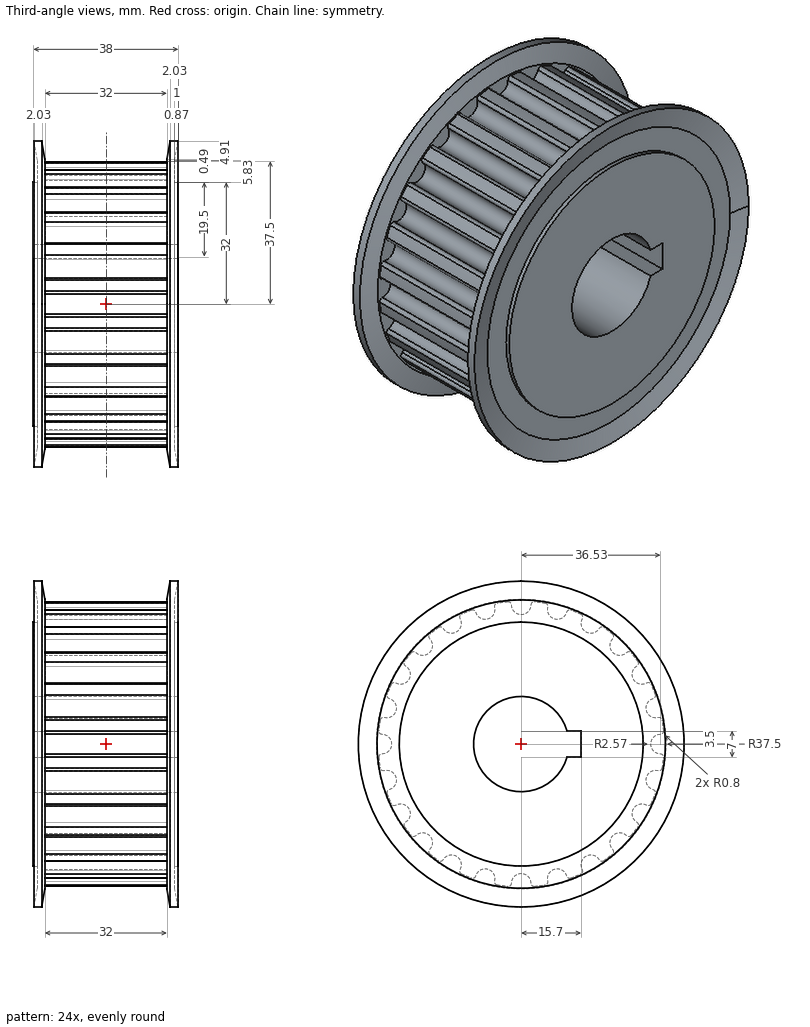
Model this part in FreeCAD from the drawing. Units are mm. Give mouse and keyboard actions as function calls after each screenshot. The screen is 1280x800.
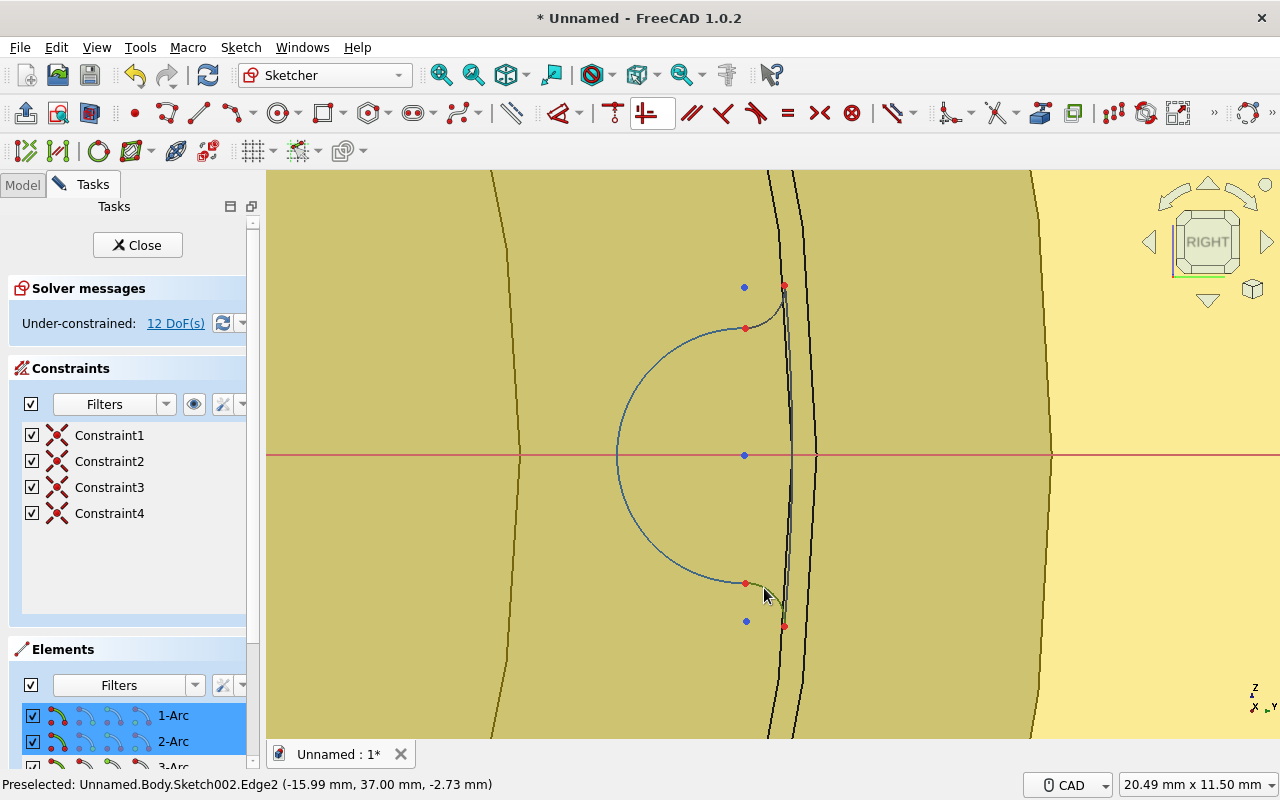
click(756, 114)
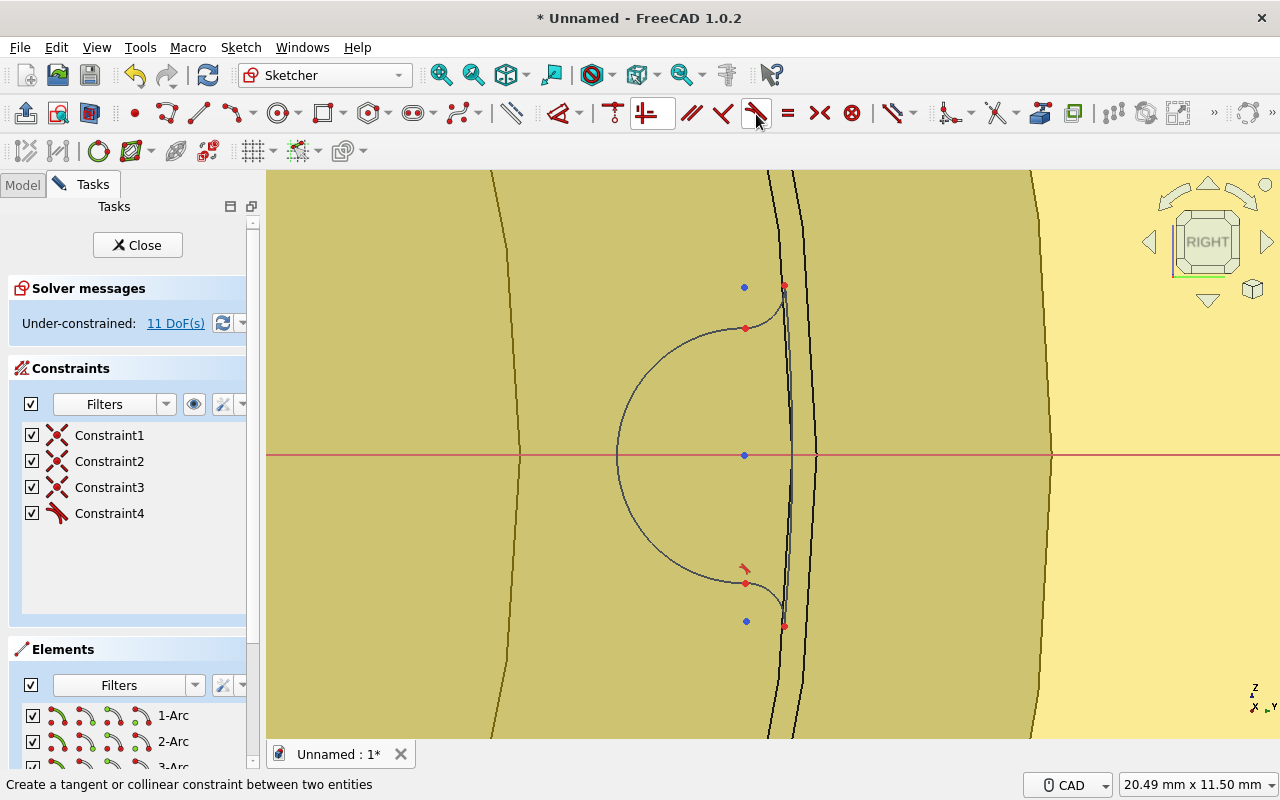
click(641, 381)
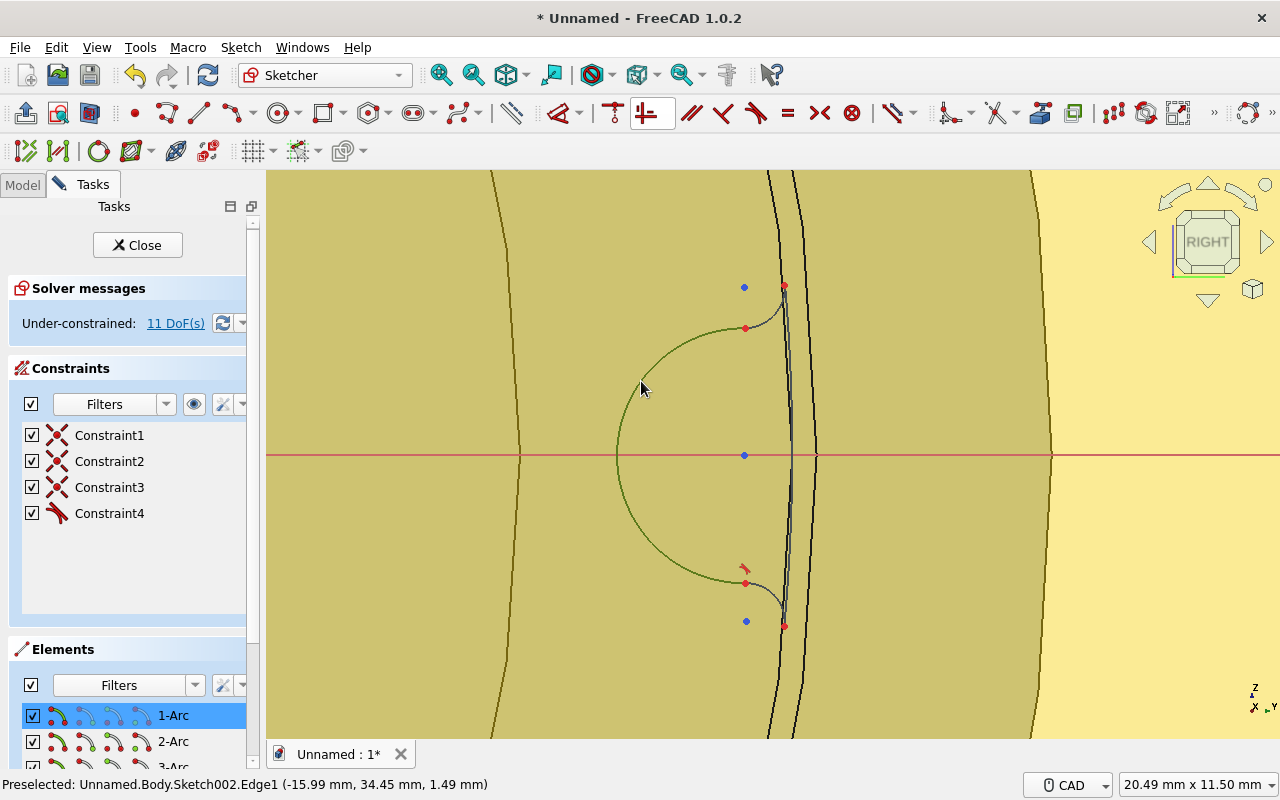
click(764, 323)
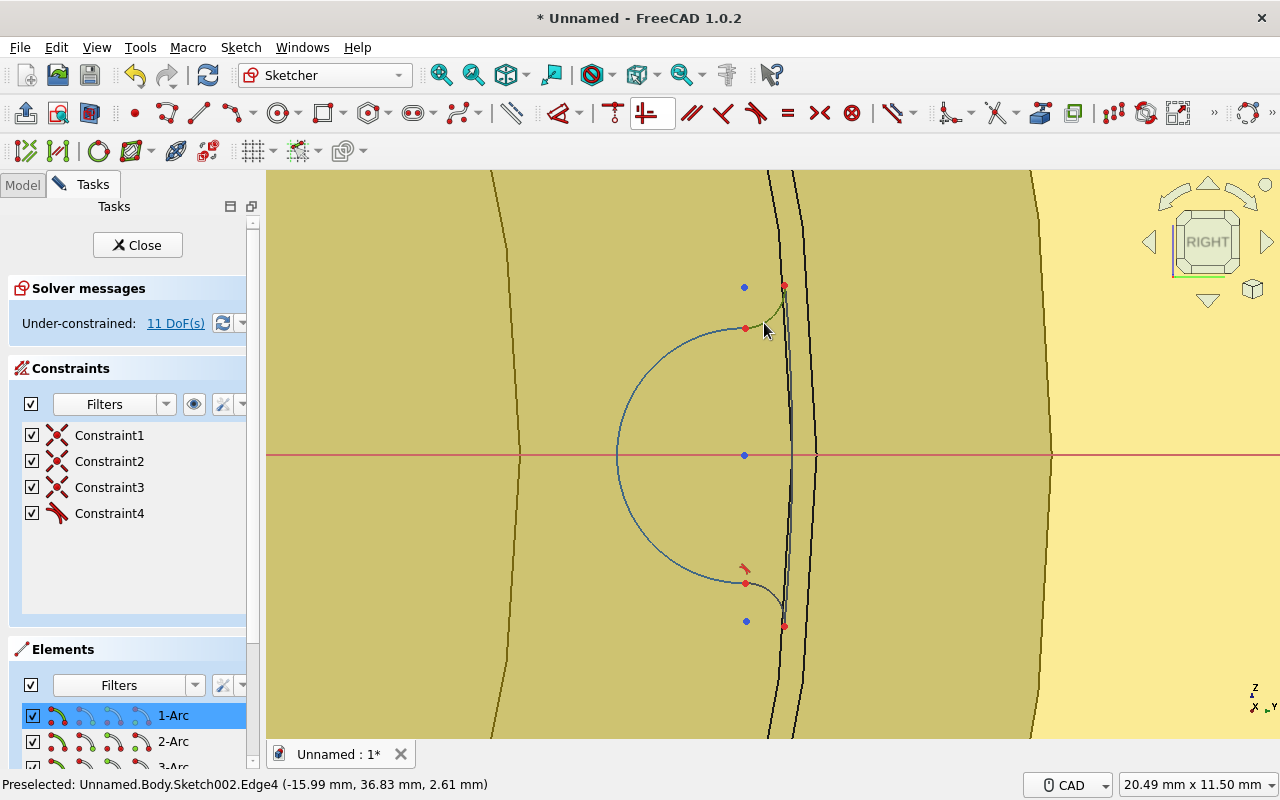
click(756, 114)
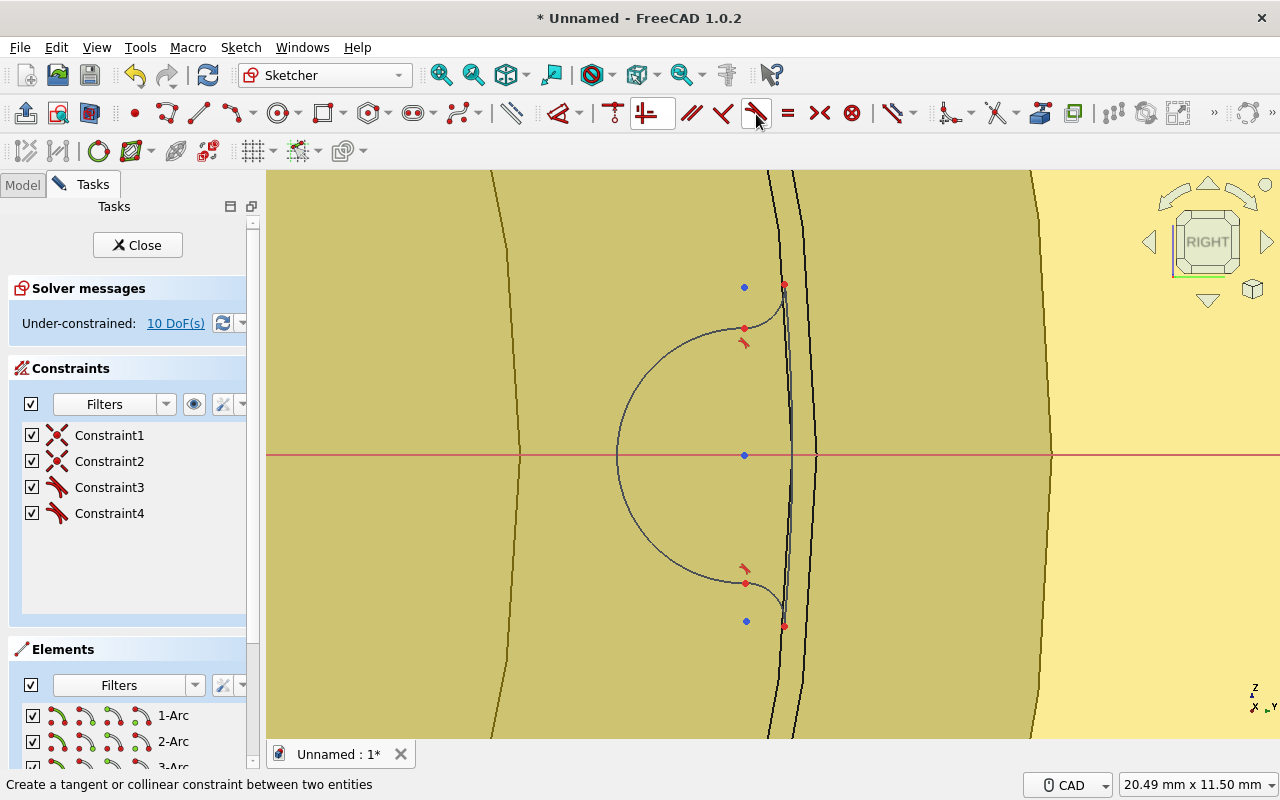
click(765, 588)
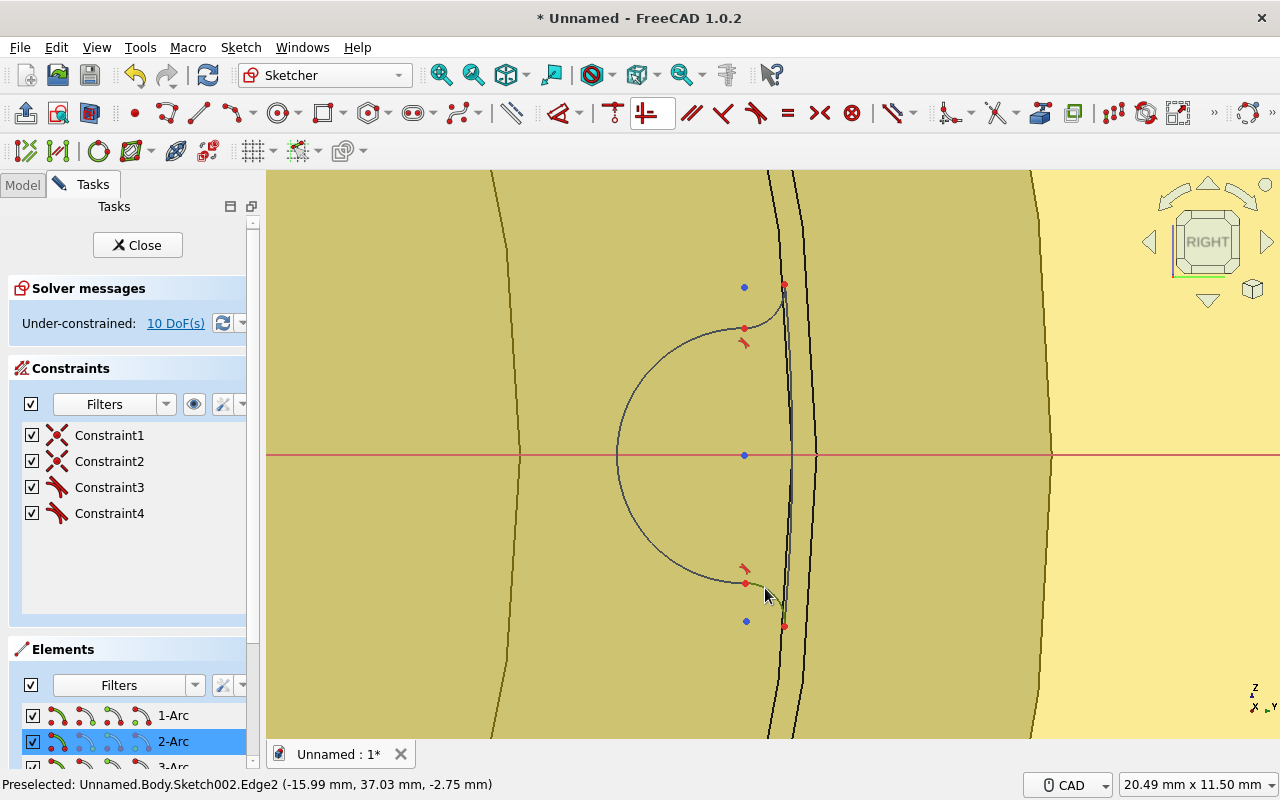
click(791, 524)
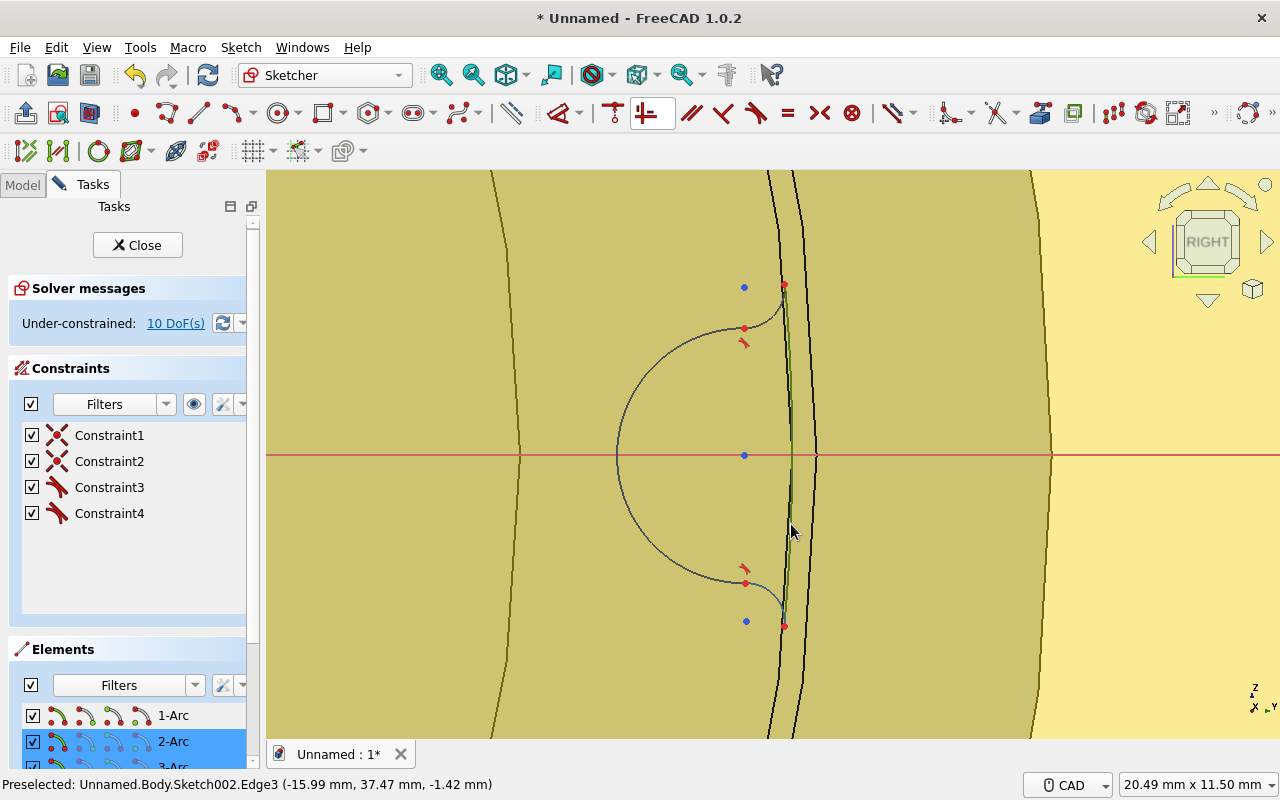
click(756, 114)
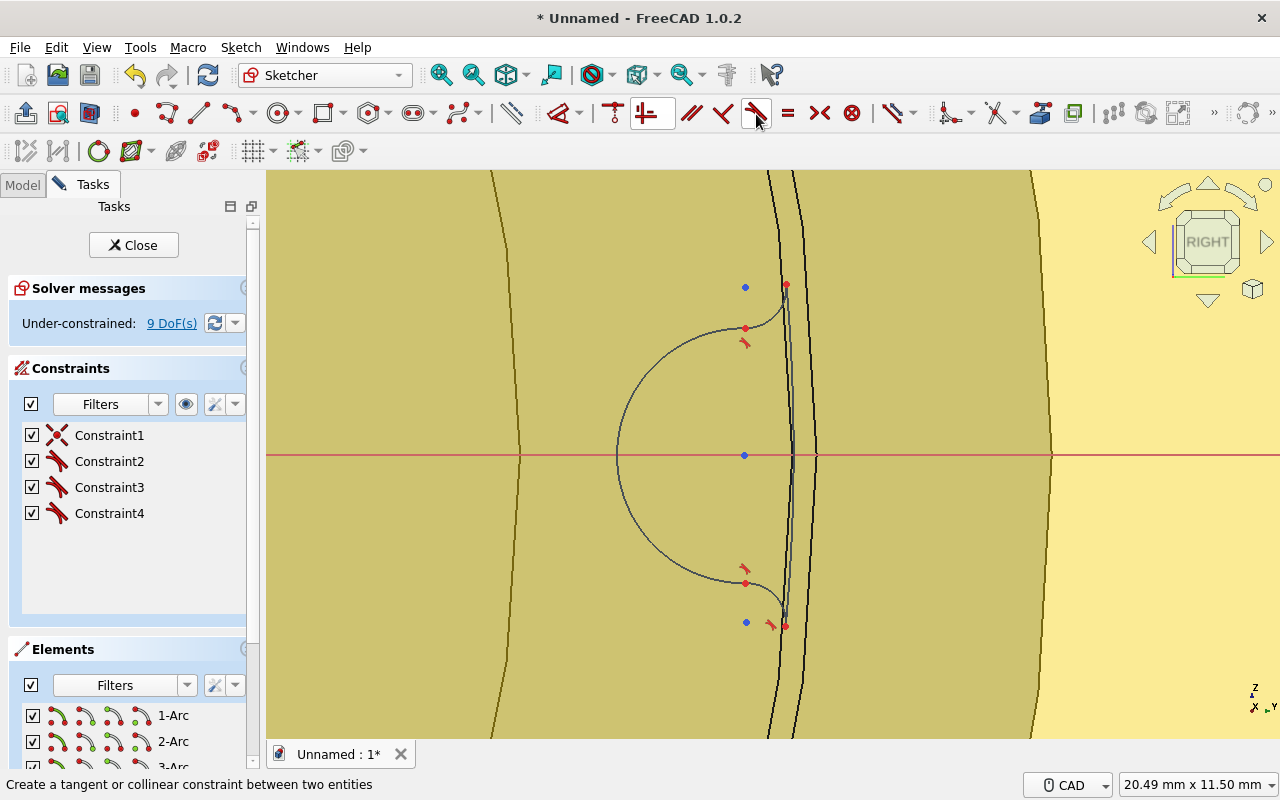
click(792, 524)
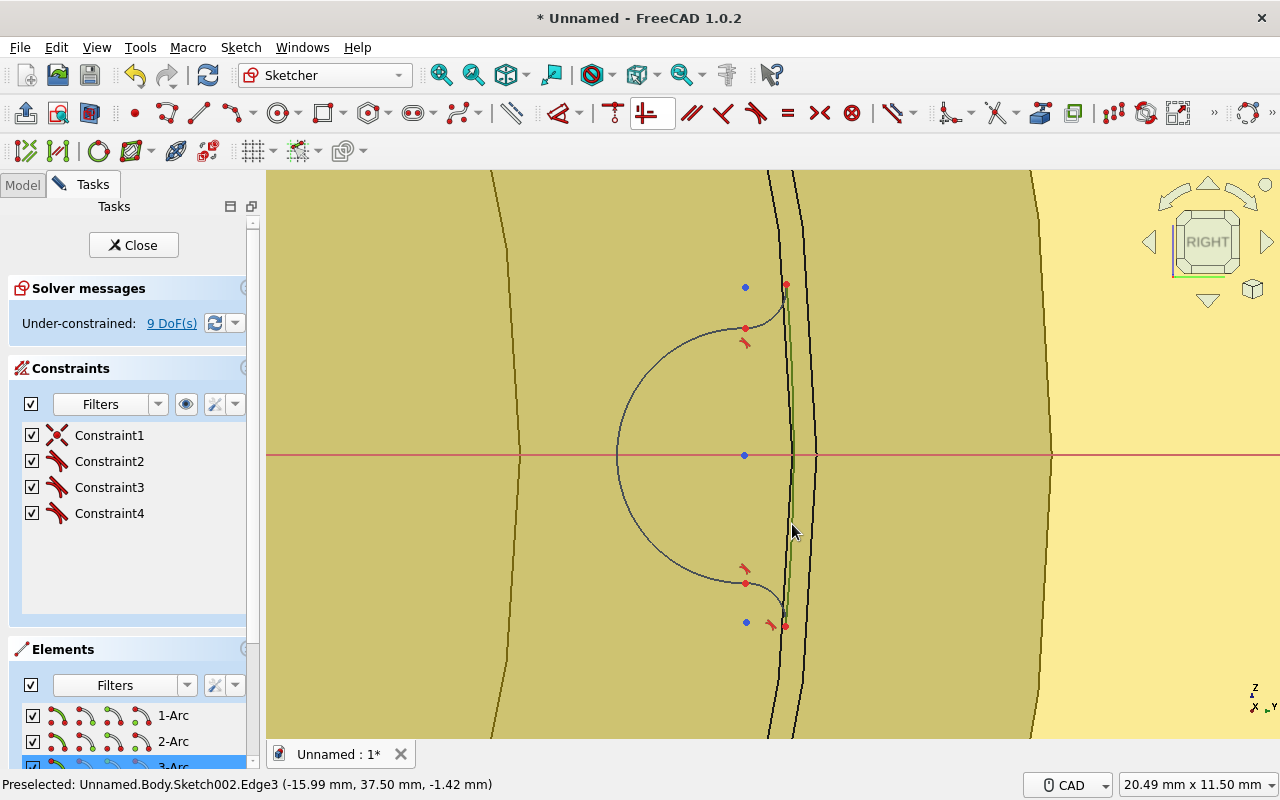
click(765, 324)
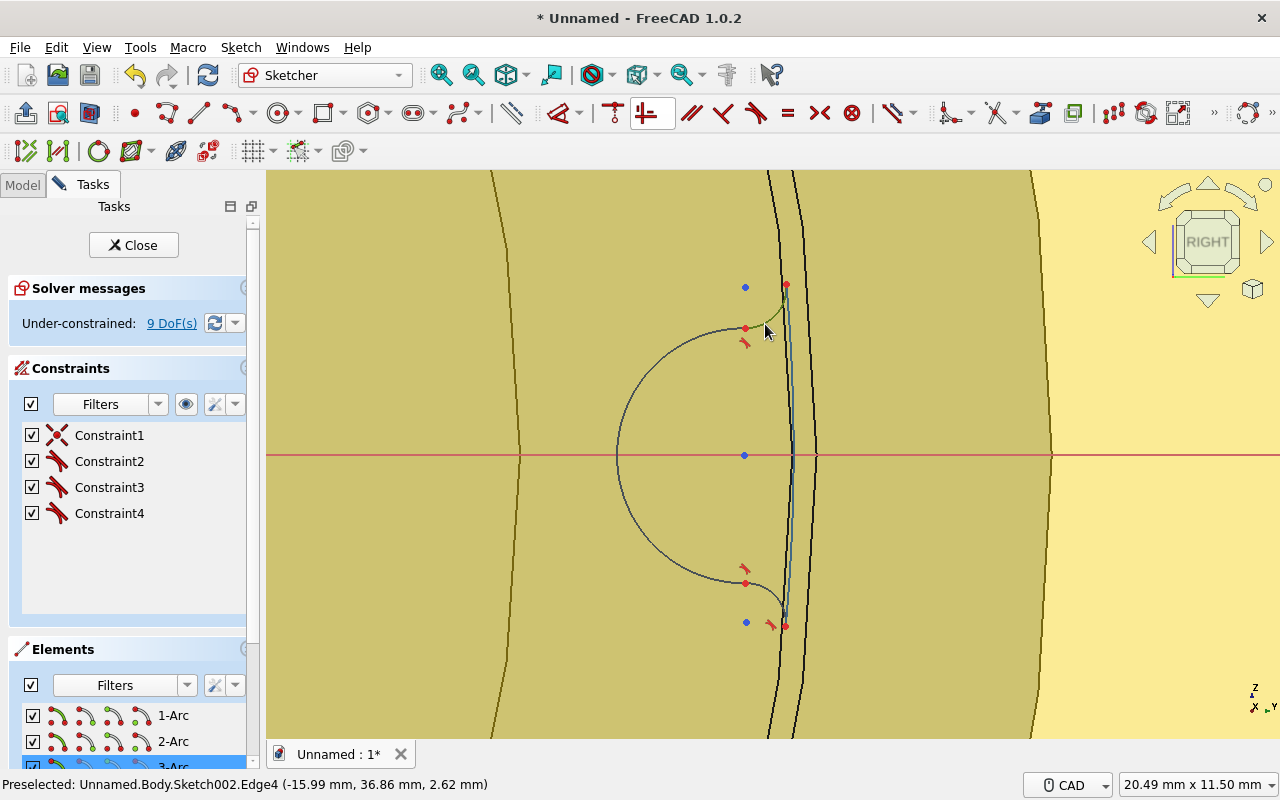
click(756, 114)